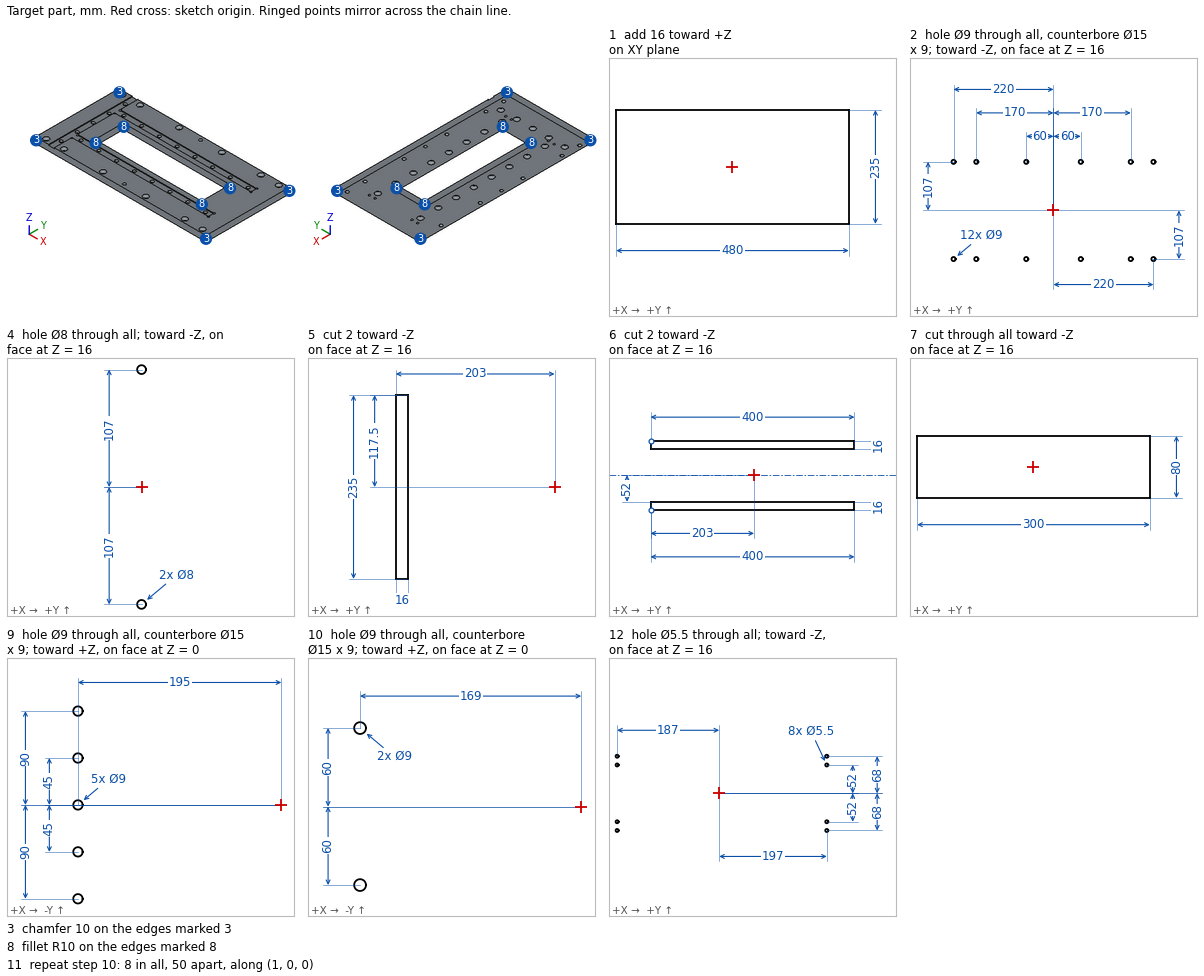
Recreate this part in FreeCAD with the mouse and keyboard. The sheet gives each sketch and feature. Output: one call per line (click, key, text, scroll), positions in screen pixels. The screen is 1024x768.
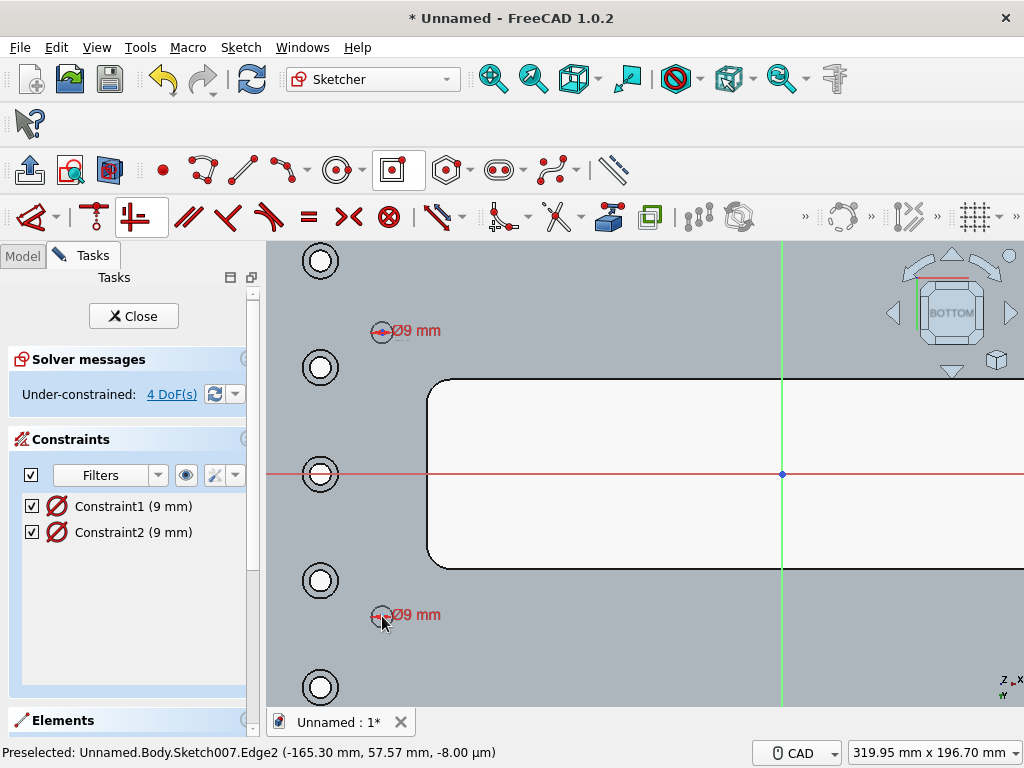
click(382, 333)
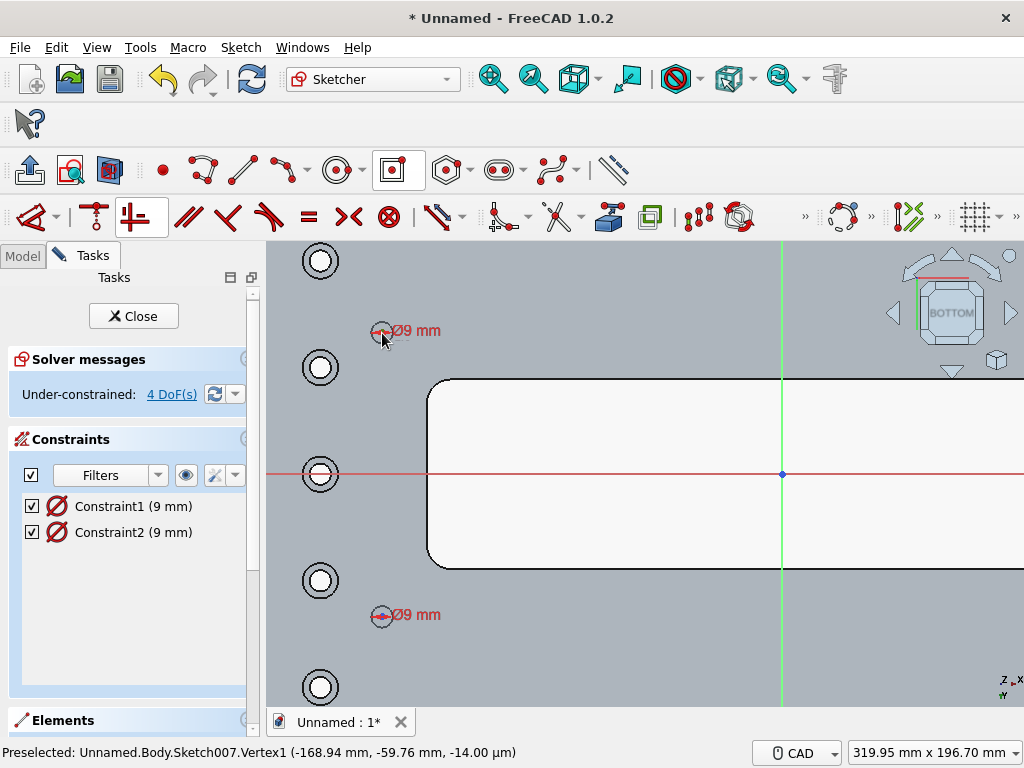
click(382, 617)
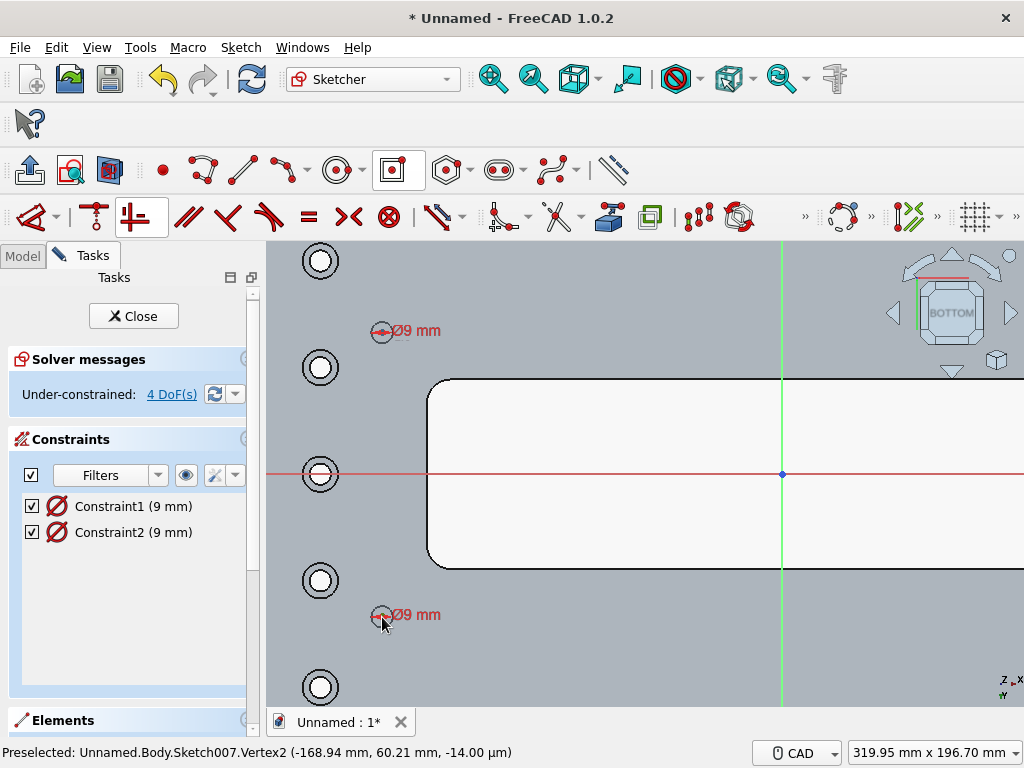
key(v)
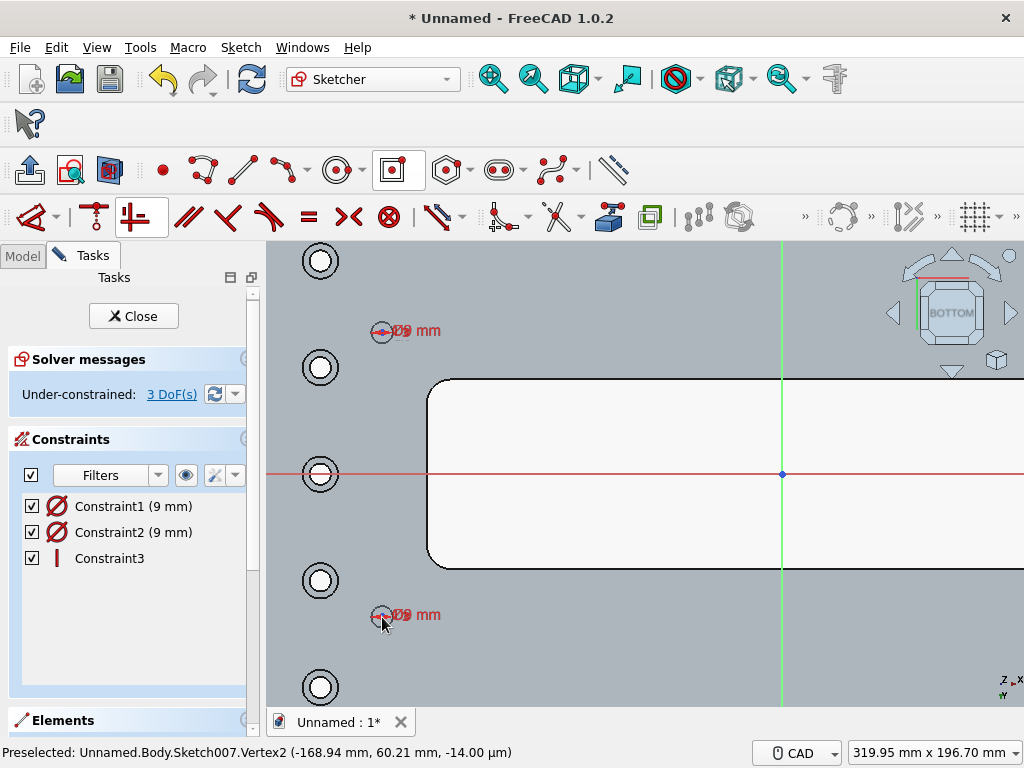
click(32, 218)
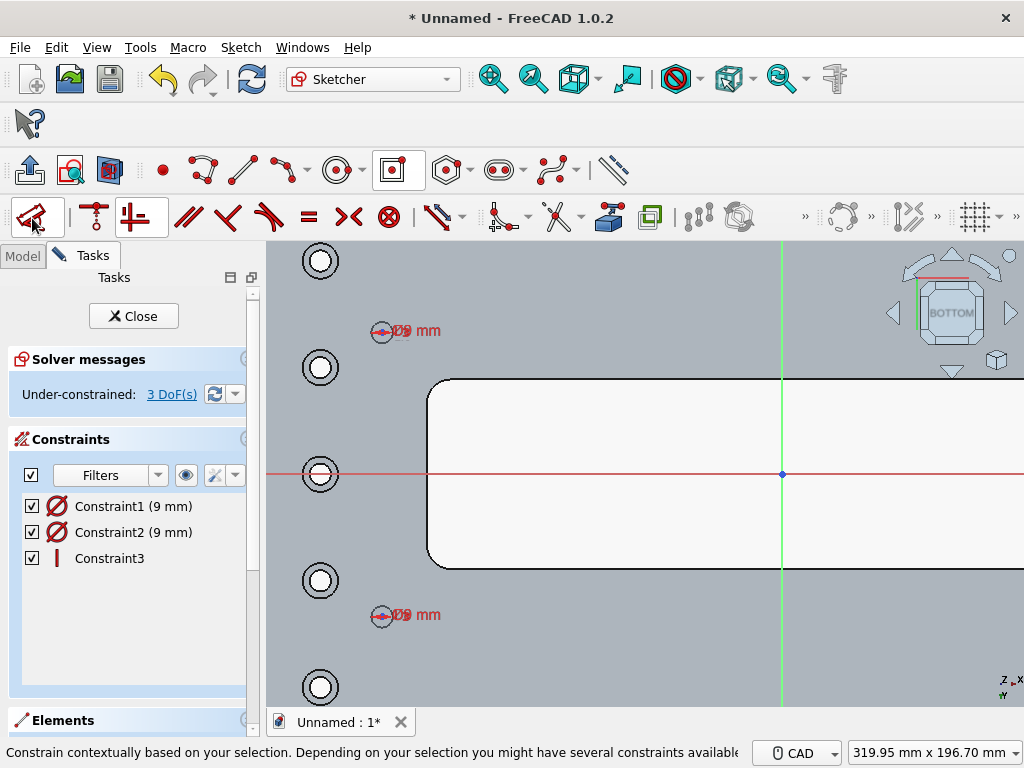
click(382, 333)
click(816, 403)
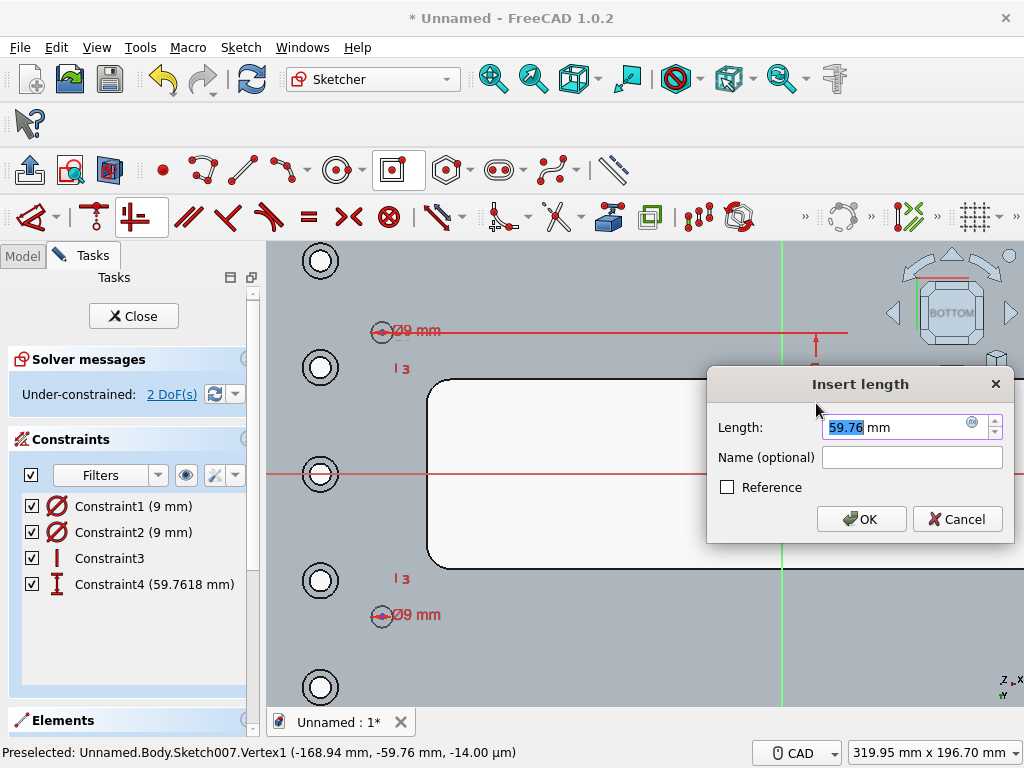
text(60)
key(Return)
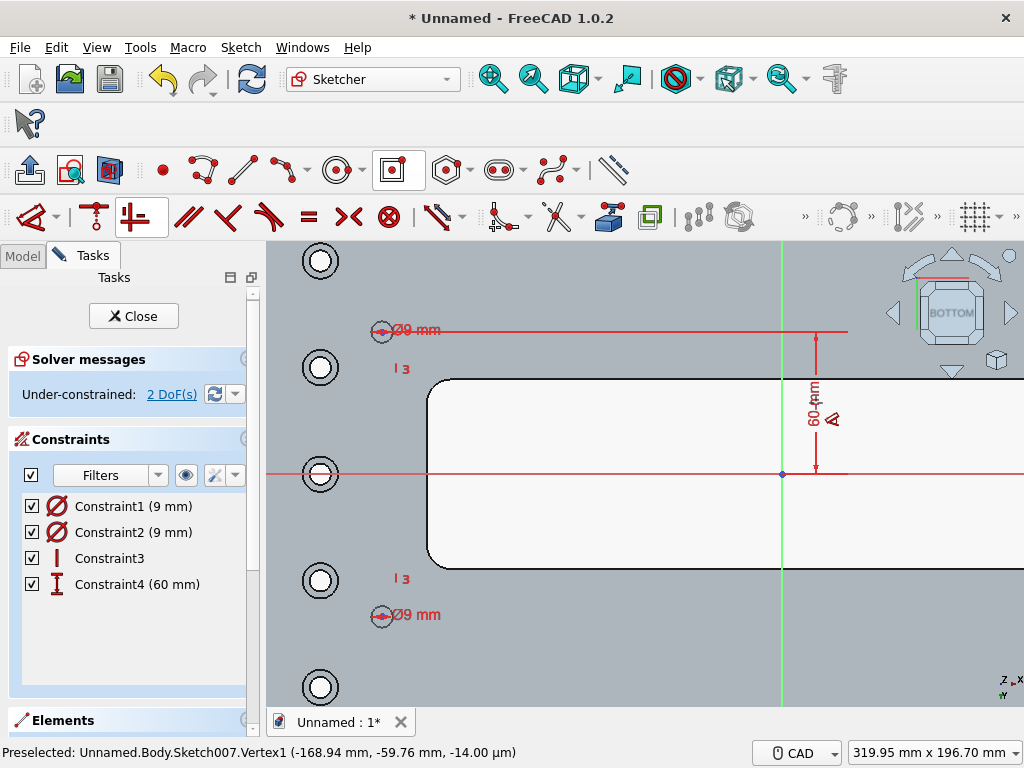
click(382, 617)
click(816, 546)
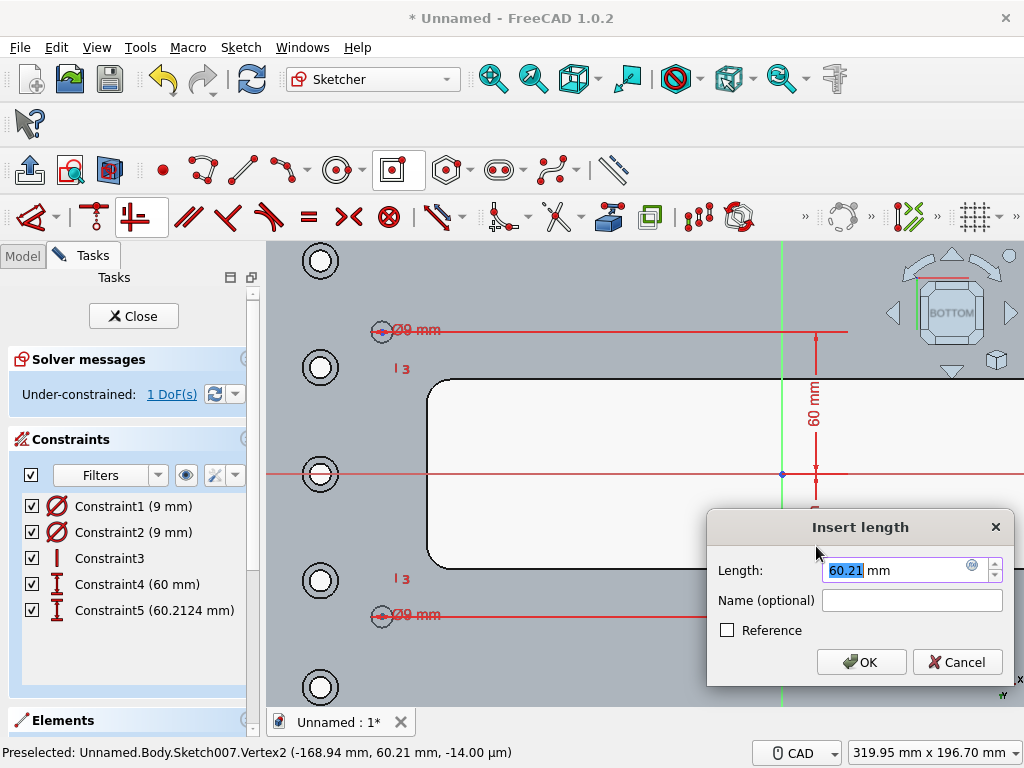
text(60)
key(Return)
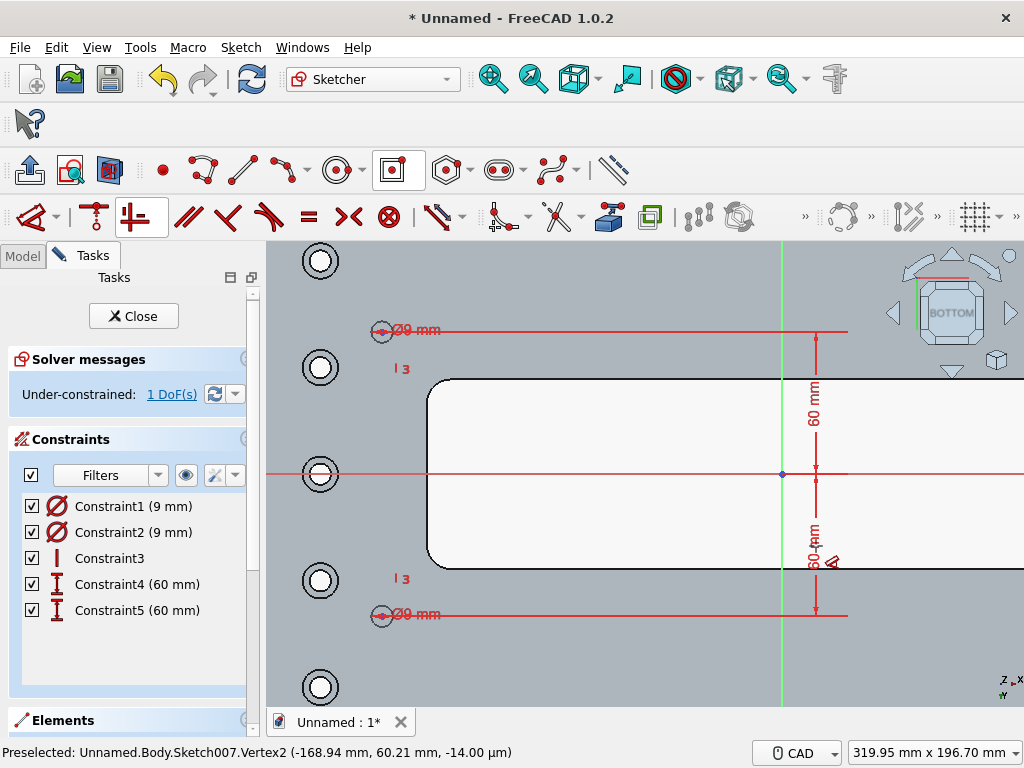
click(382, 332)
click(582, 298)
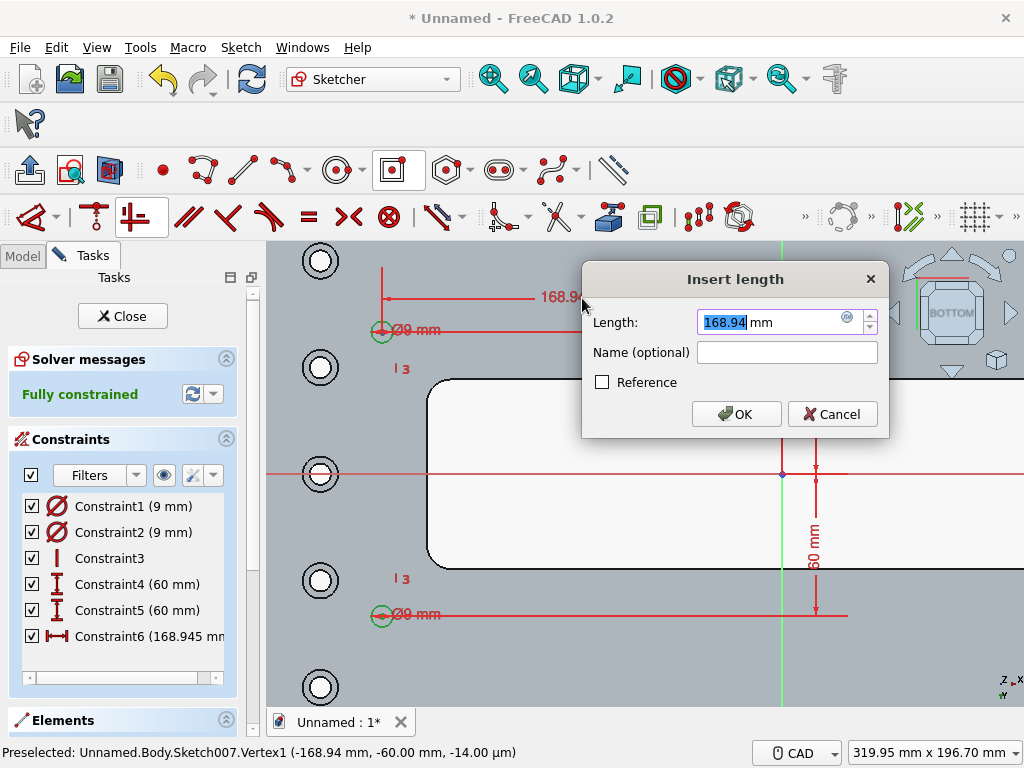
text(169)
key(Return)
key(Escape)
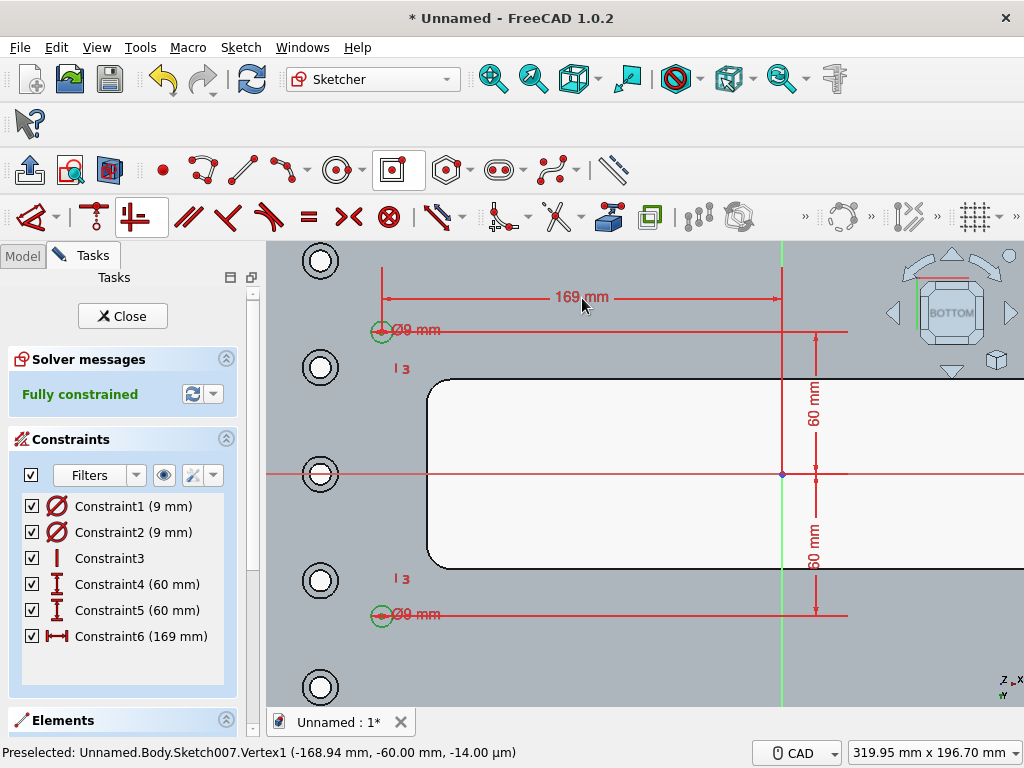
click(123, 316)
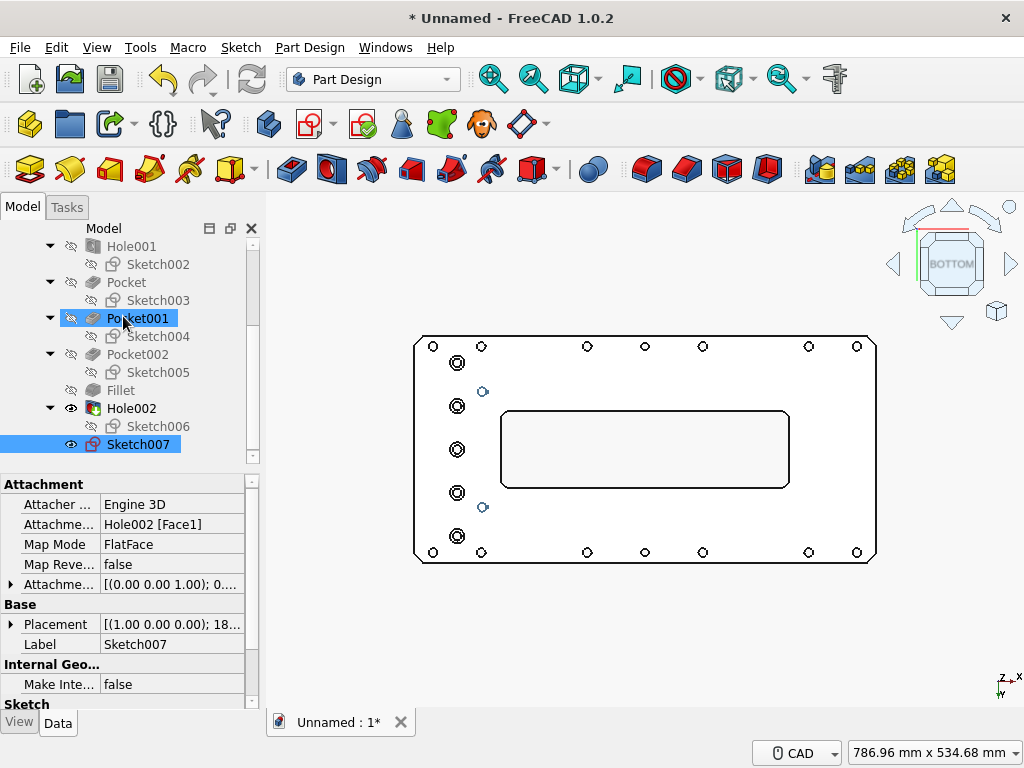
click(332, 170)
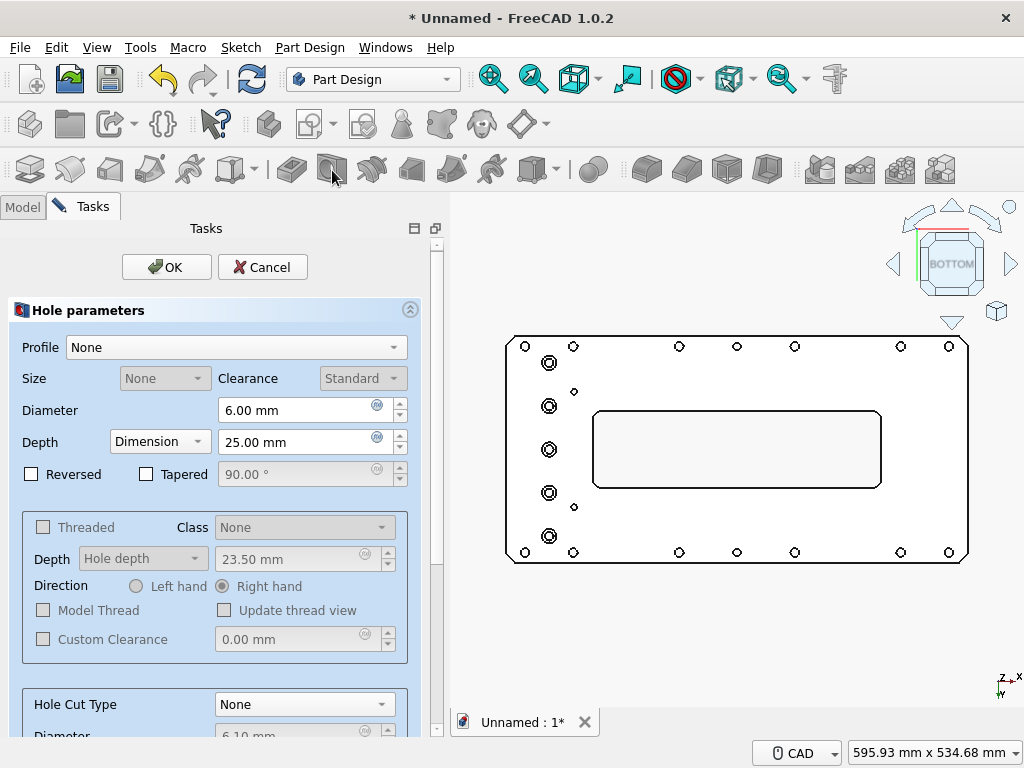
triple_click(305, 410)